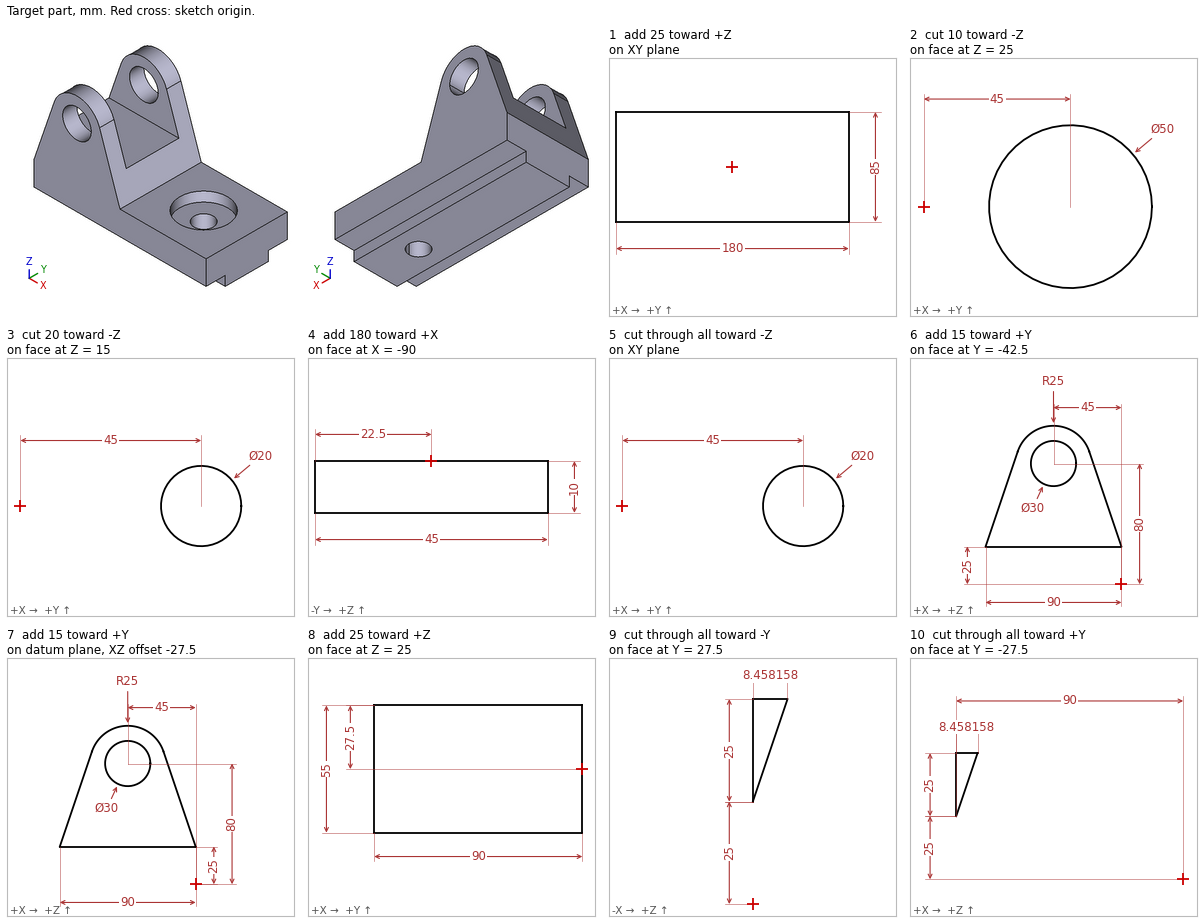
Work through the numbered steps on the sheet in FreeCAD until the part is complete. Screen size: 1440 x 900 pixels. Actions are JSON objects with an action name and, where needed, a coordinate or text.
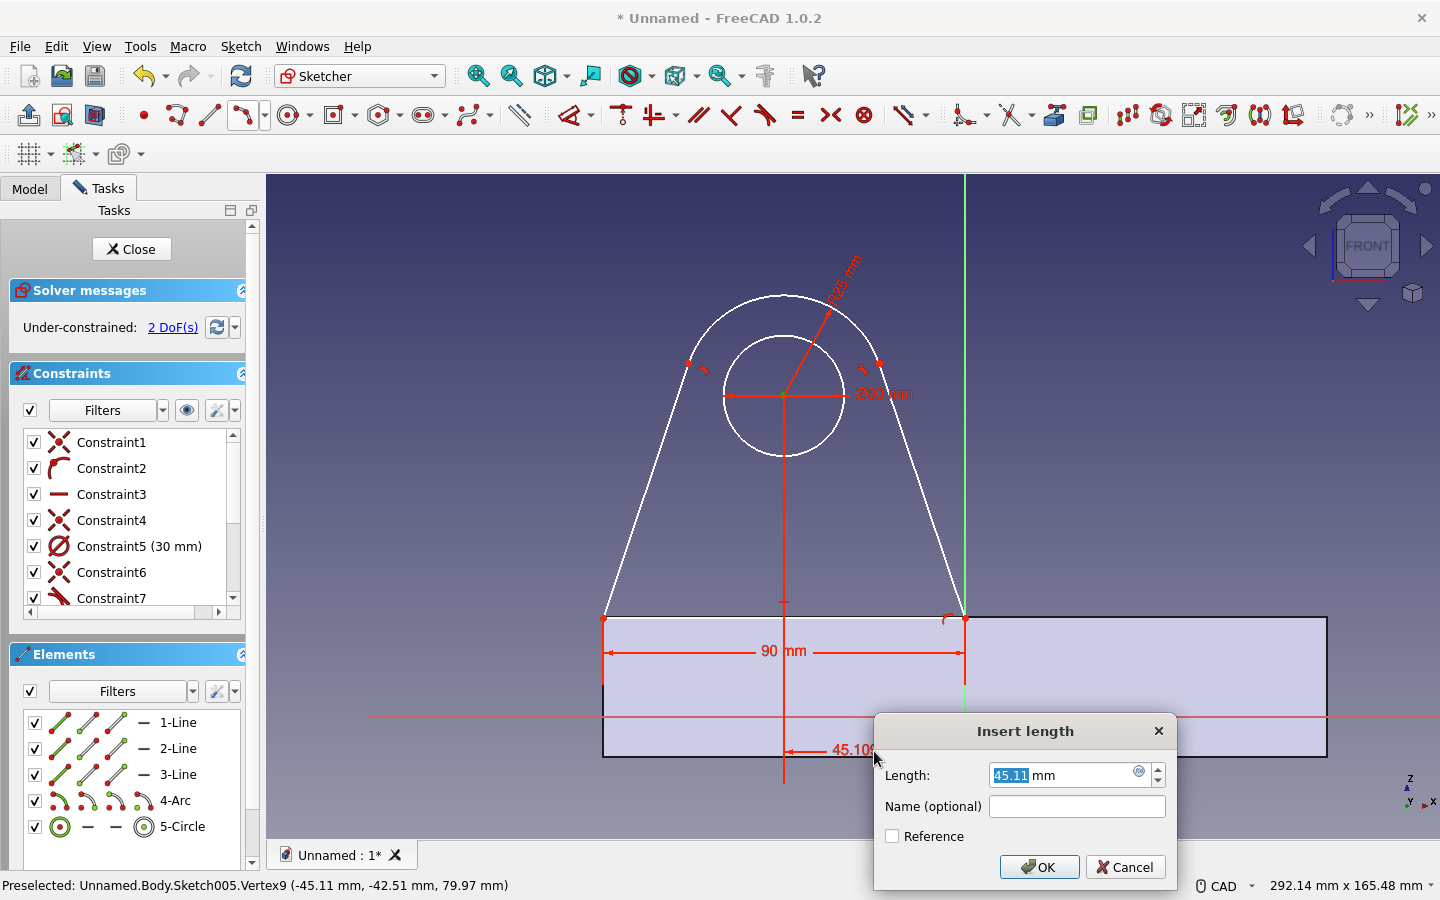
{"action": "type", "text": "45"}
{"action": "key", "text": "Return"}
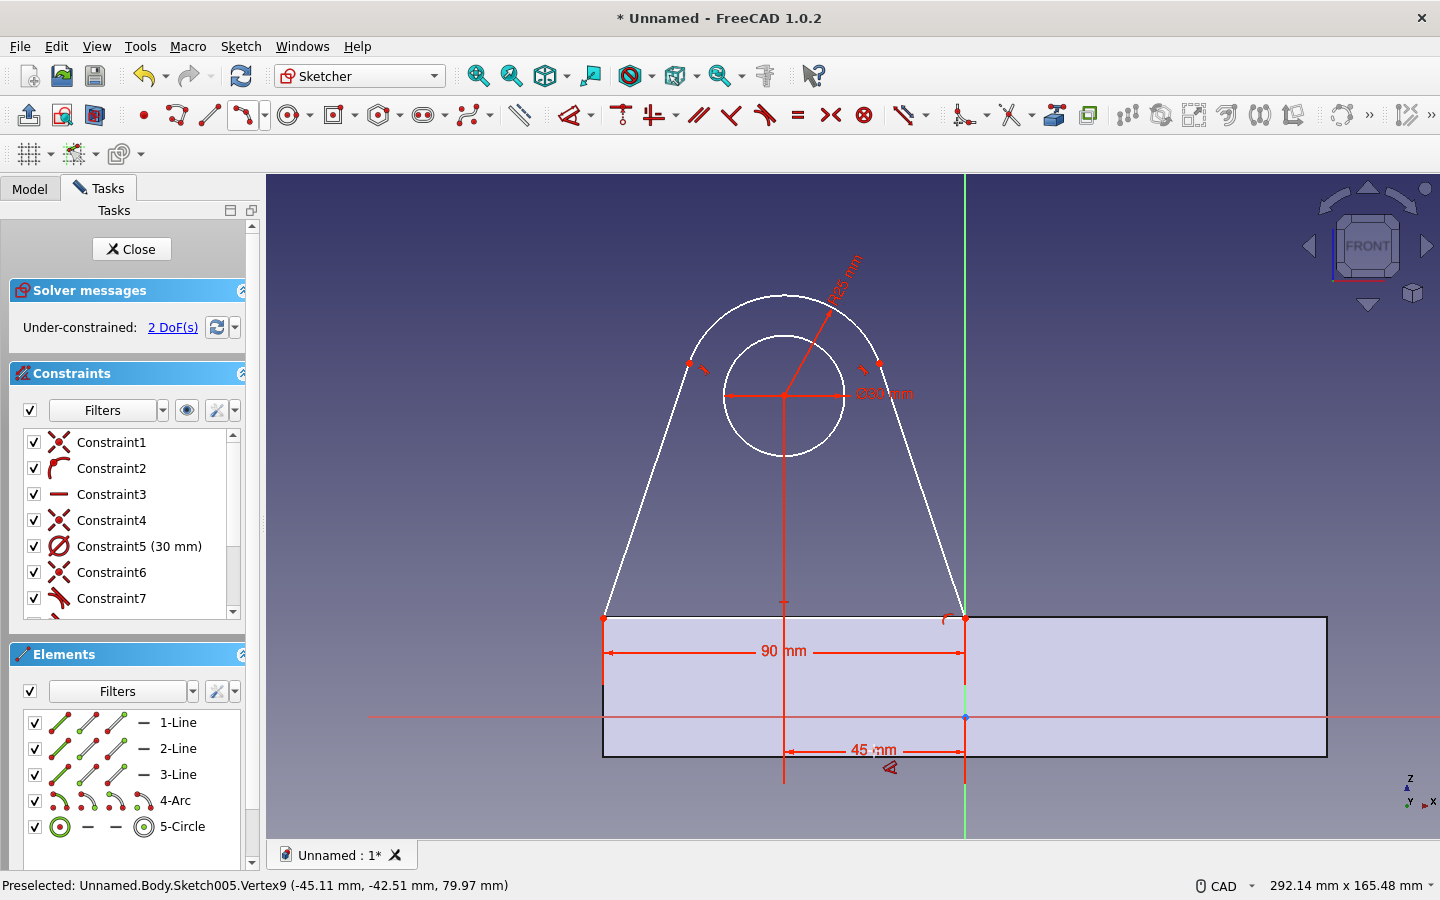
{"action": "left_click", "coordinate": [784, 396]}
{"action": "left_click", "coordinate": [999, 557]}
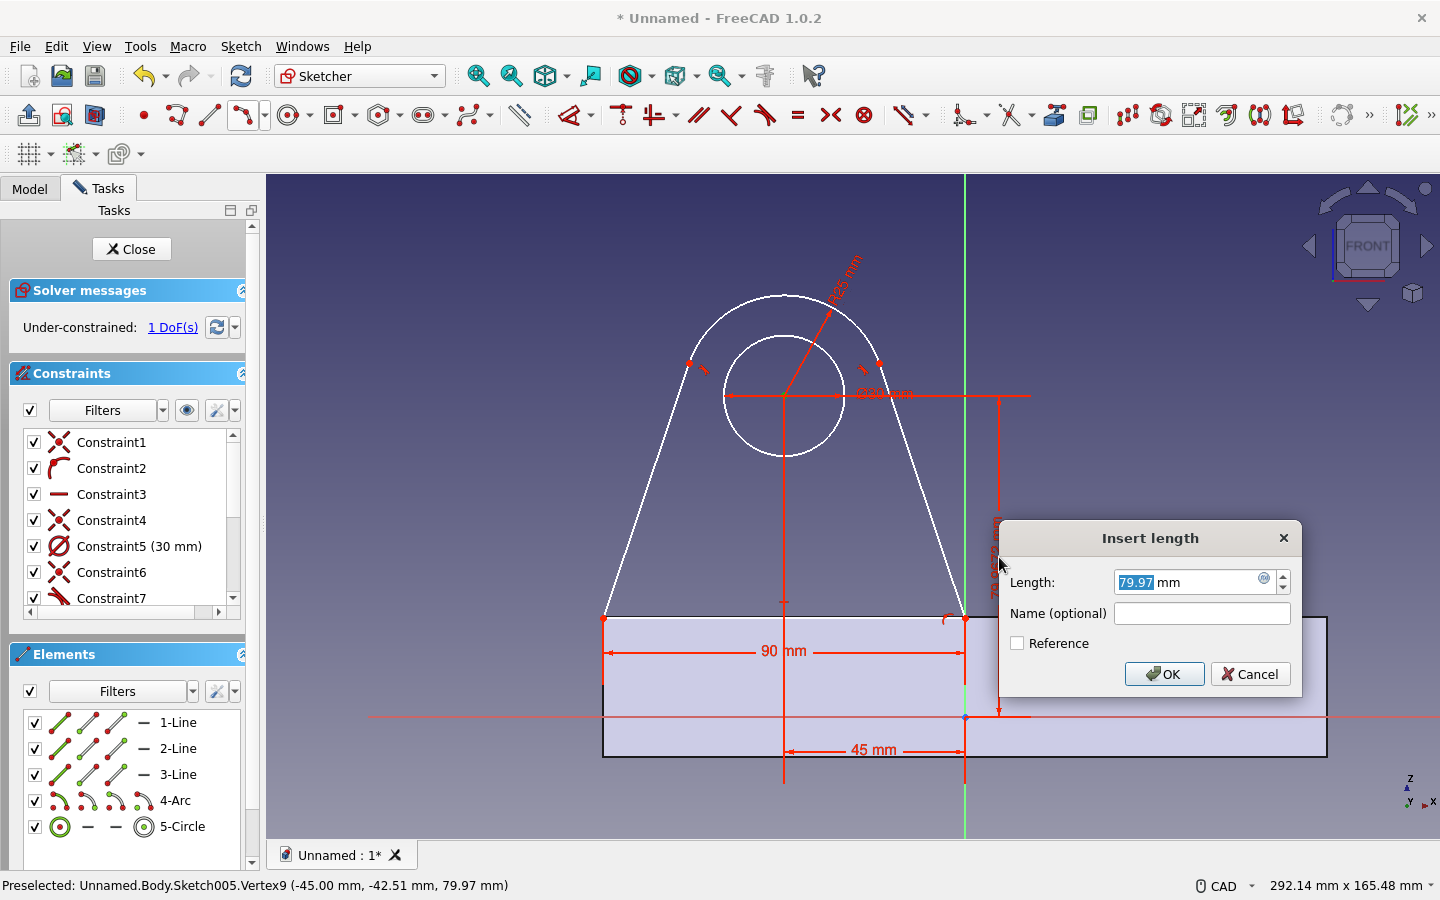
{"action": "type", "text": "80"}
{"action": "key", "text": "Return"}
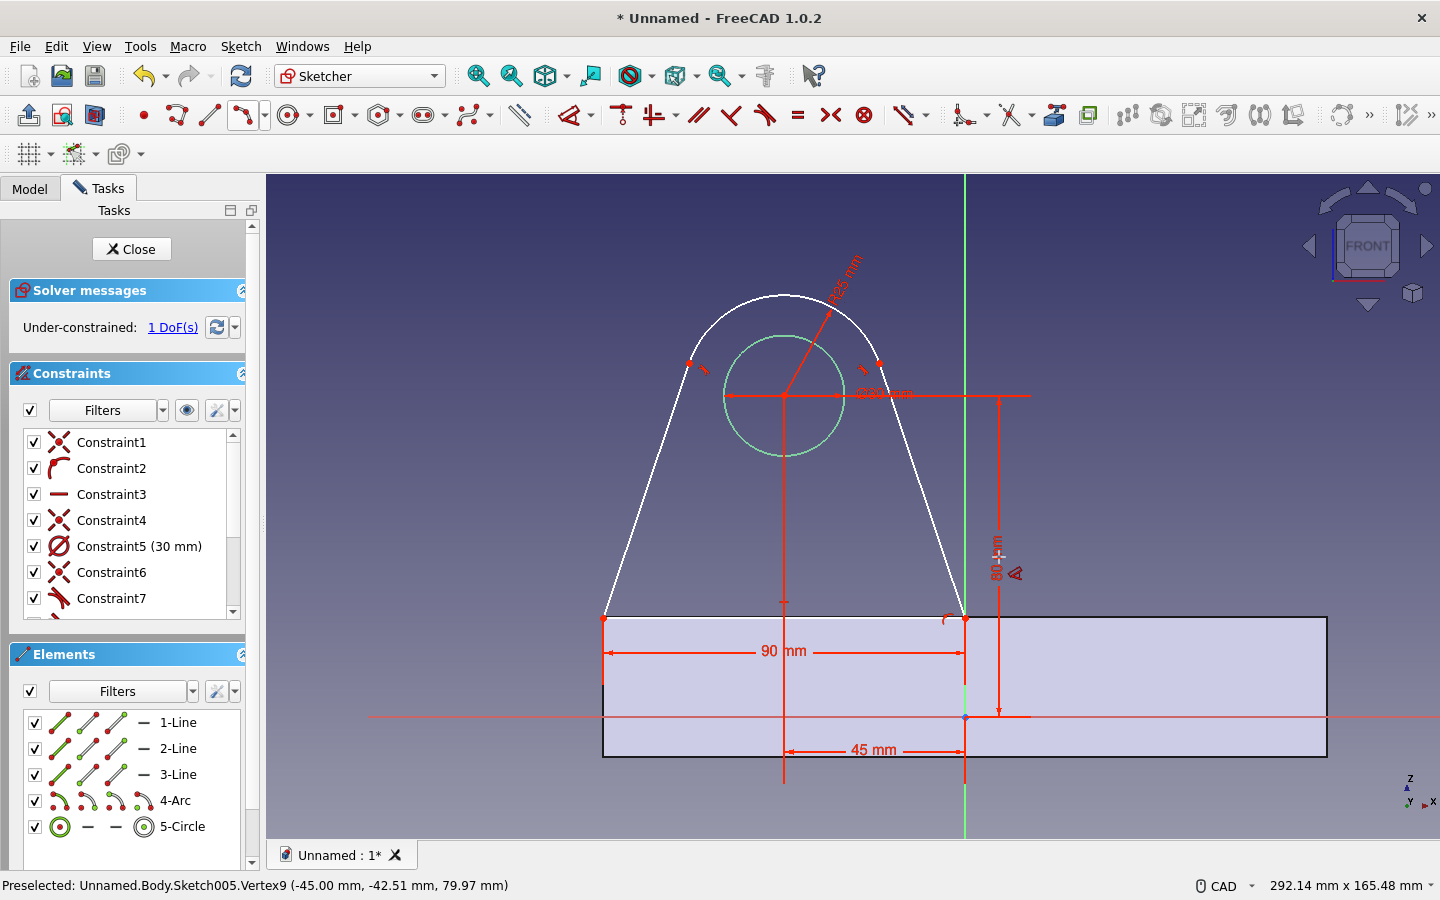
{"action": "left_click", "coordinate": [603, 618]}
{"action": "left_click", "coordinate": [999, 668]}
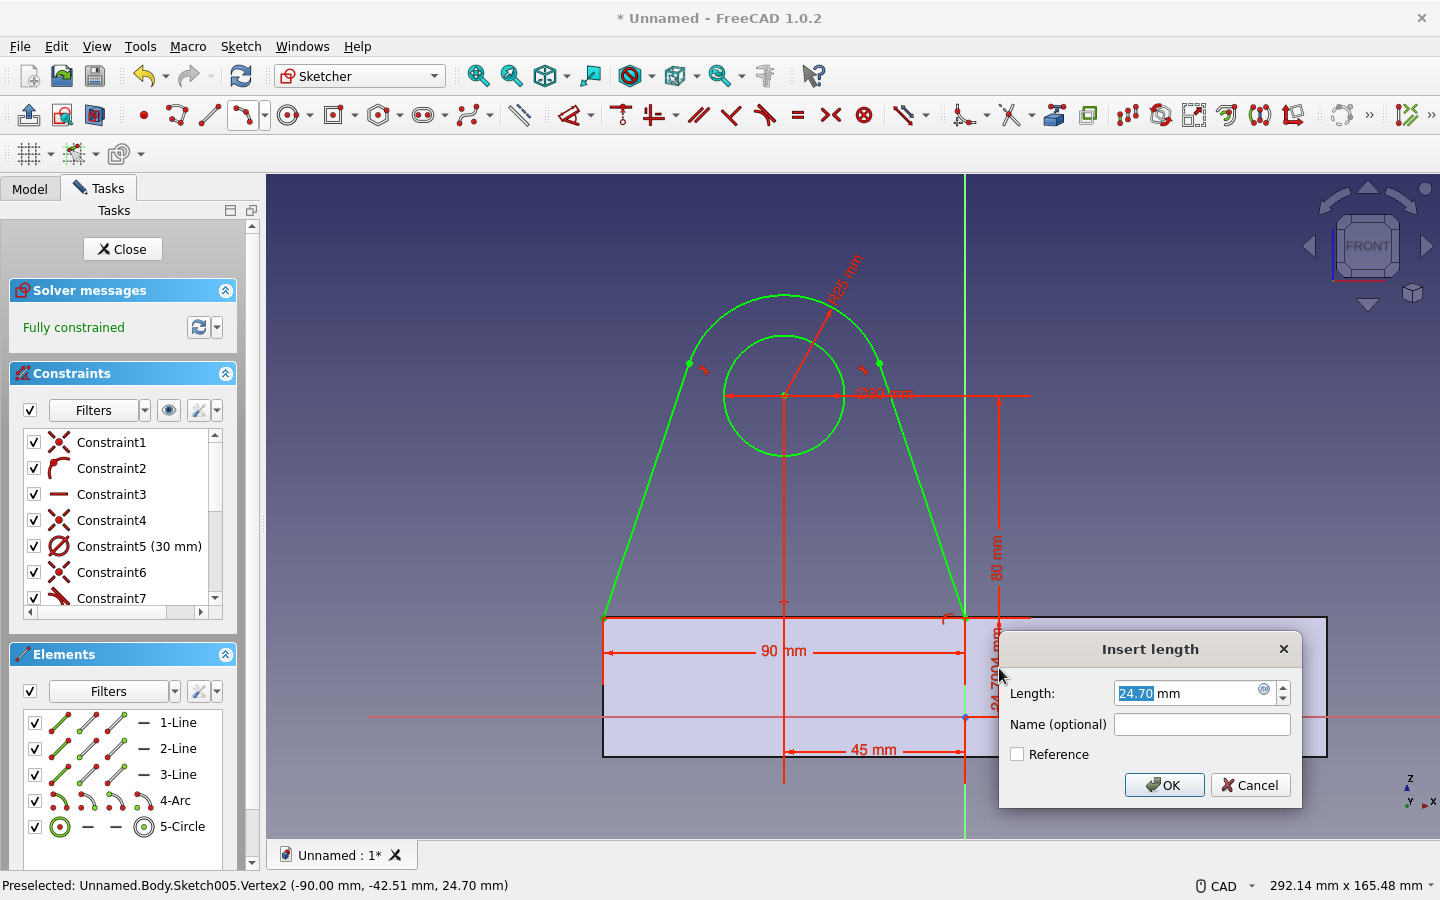
{"action": "type", "text": "25"}
{"action": "key", "text": "Return"}
{"action": "key", "text": "Escape"}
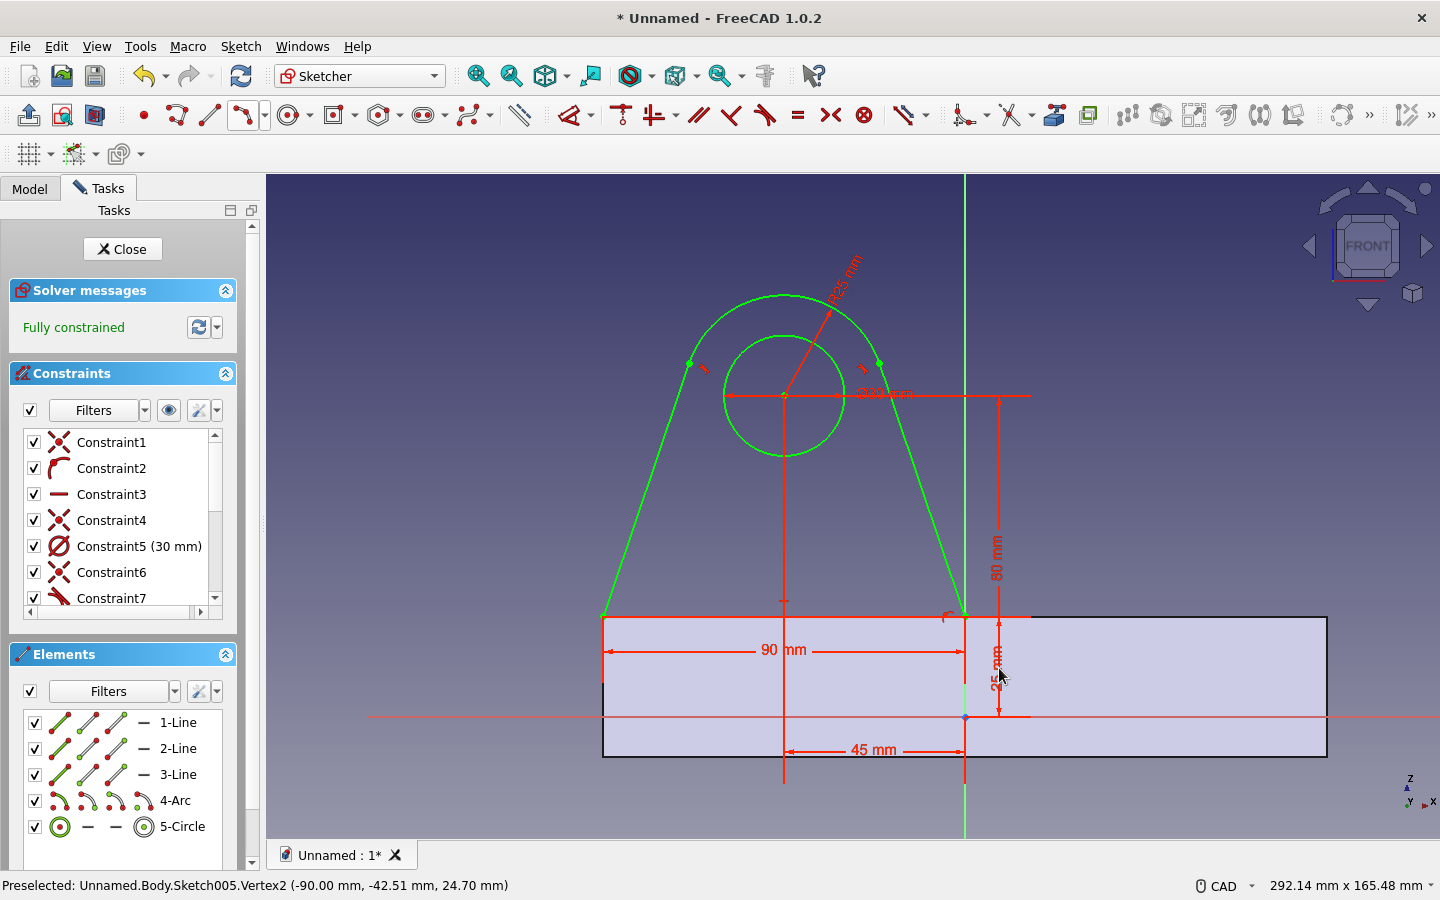
{"action": "left_click", "coordinate": [123, 249]}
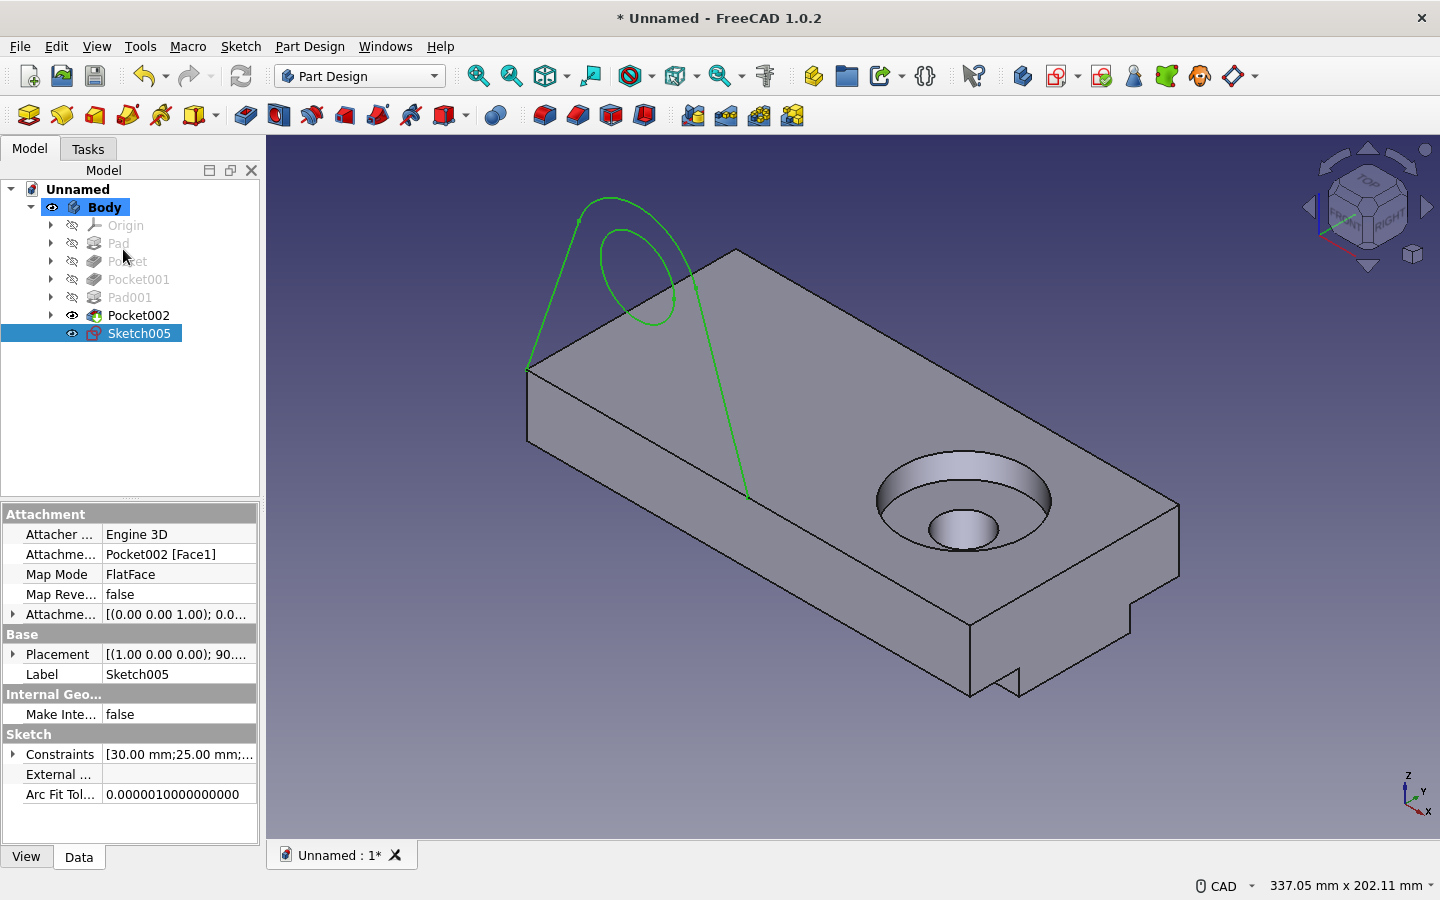
{"action": "left_click", "coordinate": [29, 116]}